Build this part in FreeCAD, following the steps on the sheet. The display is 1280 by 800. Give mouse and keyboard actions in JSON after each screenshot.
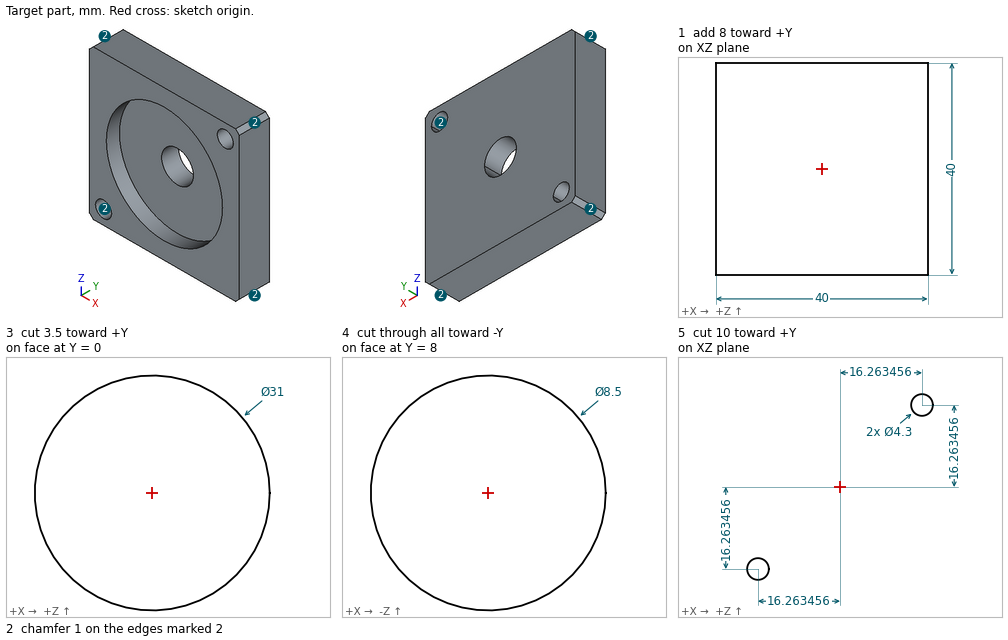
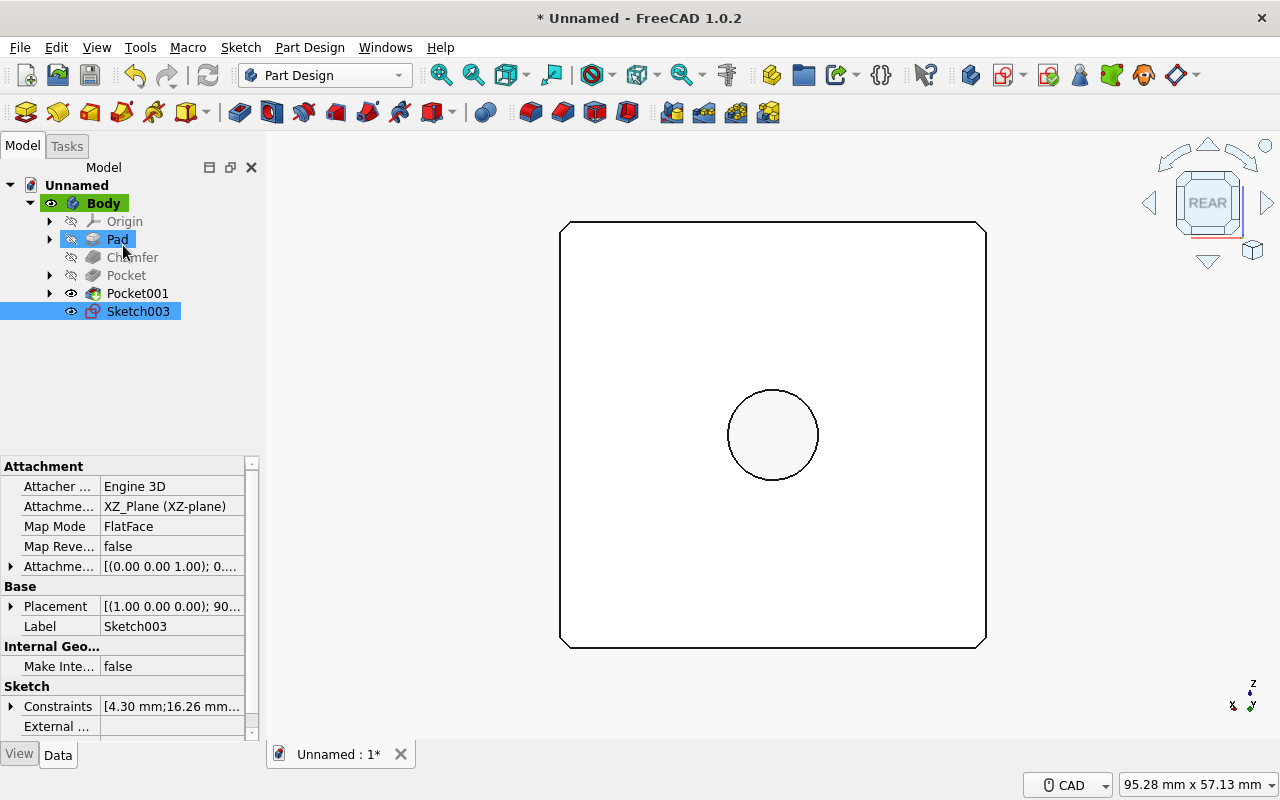
{"action": "left_click", "coordinate": [240, 112]}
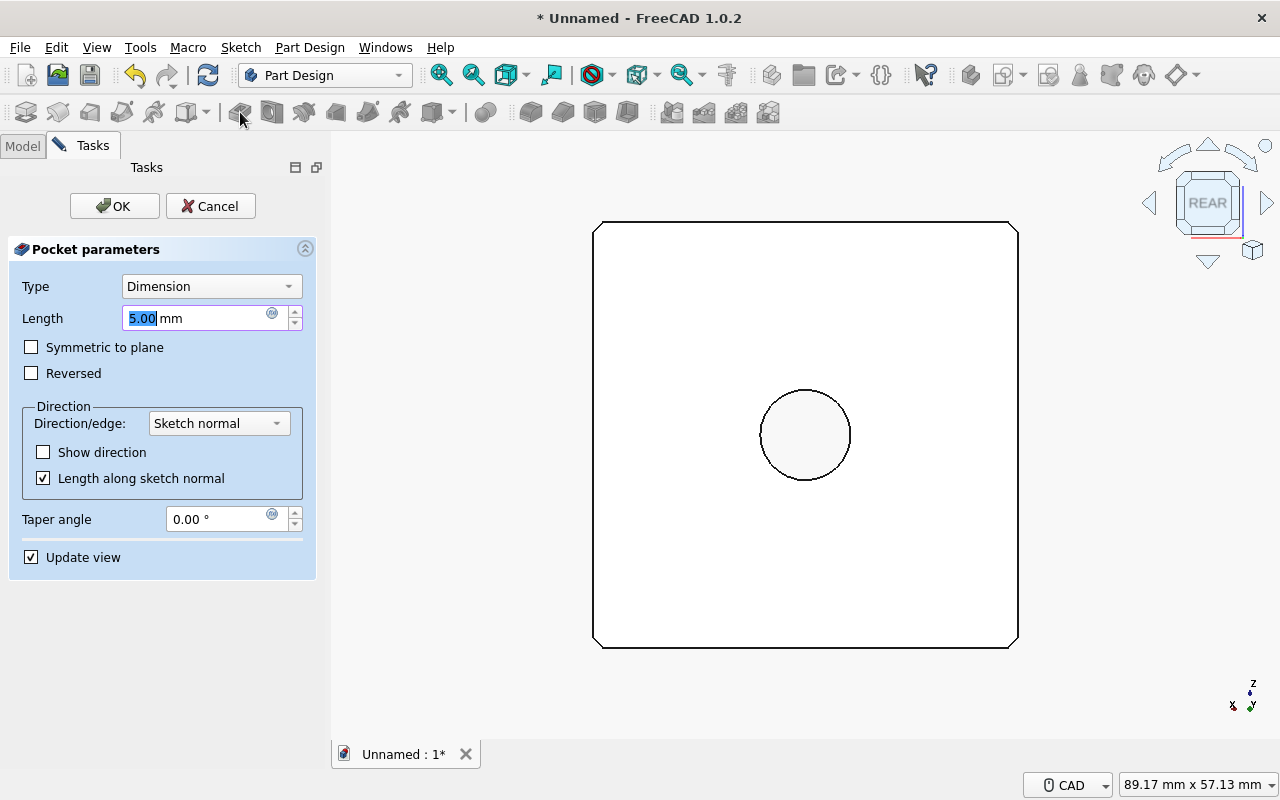
{"action": "type", "text": "10"}
{"action": "key", "text": "Tab"}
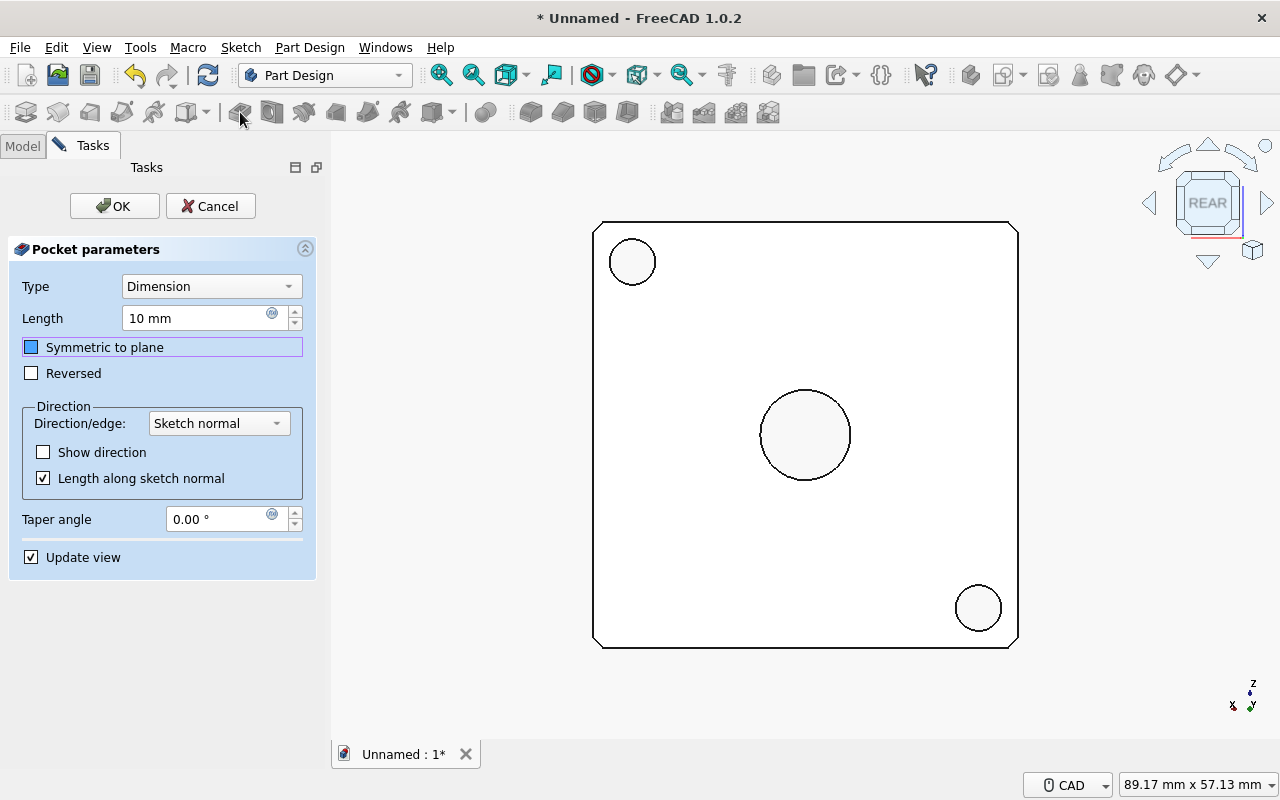
{"action": "left_click", "coordinate": [115, 206]}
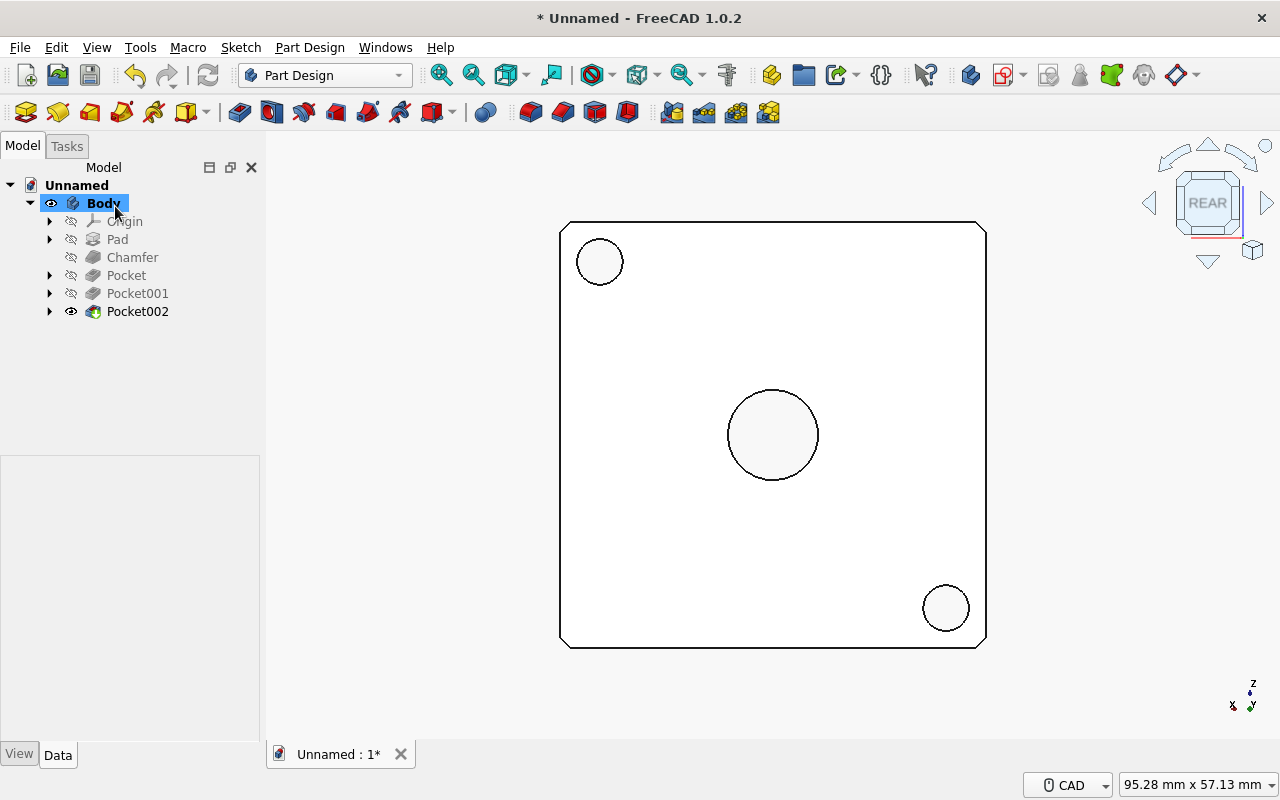
{"action": "key", "text": "0"}